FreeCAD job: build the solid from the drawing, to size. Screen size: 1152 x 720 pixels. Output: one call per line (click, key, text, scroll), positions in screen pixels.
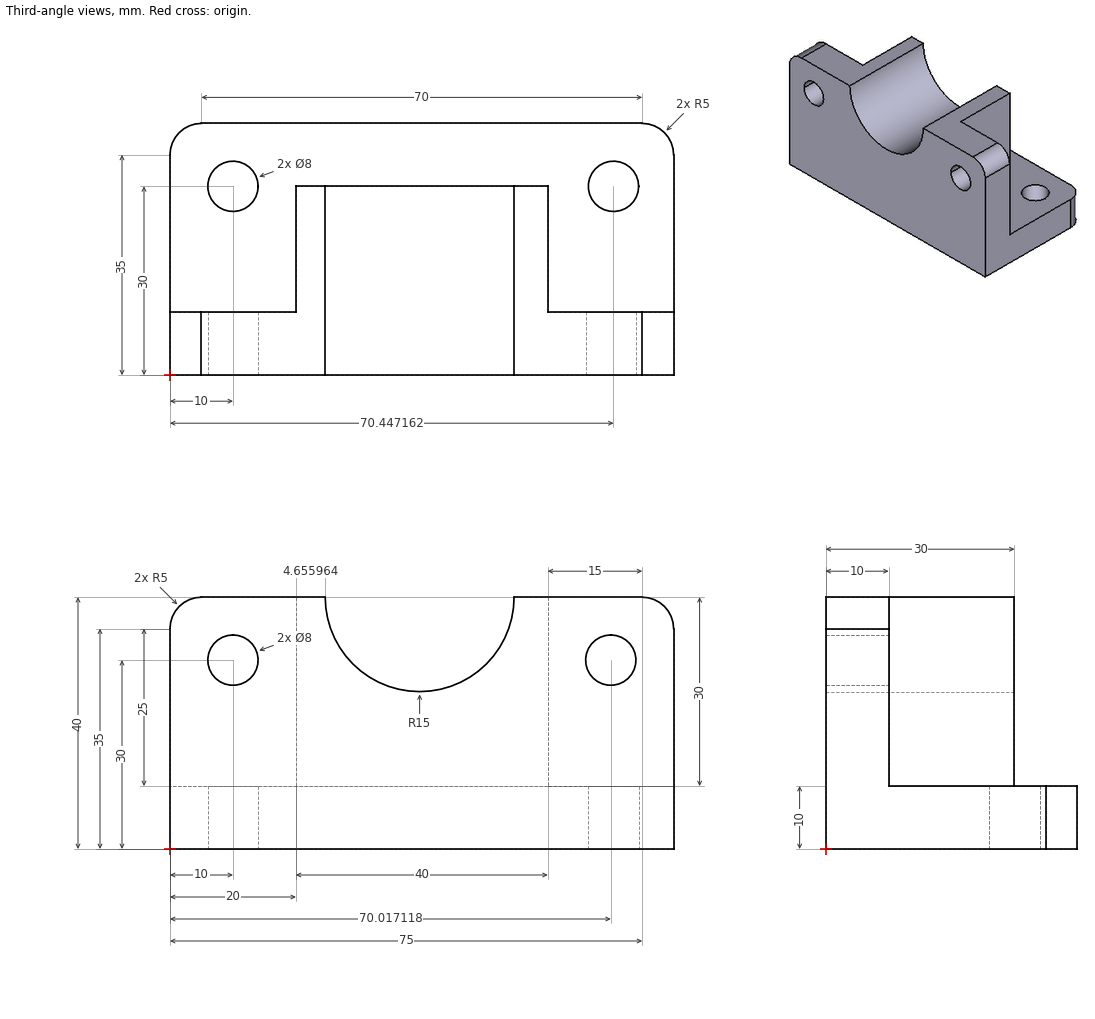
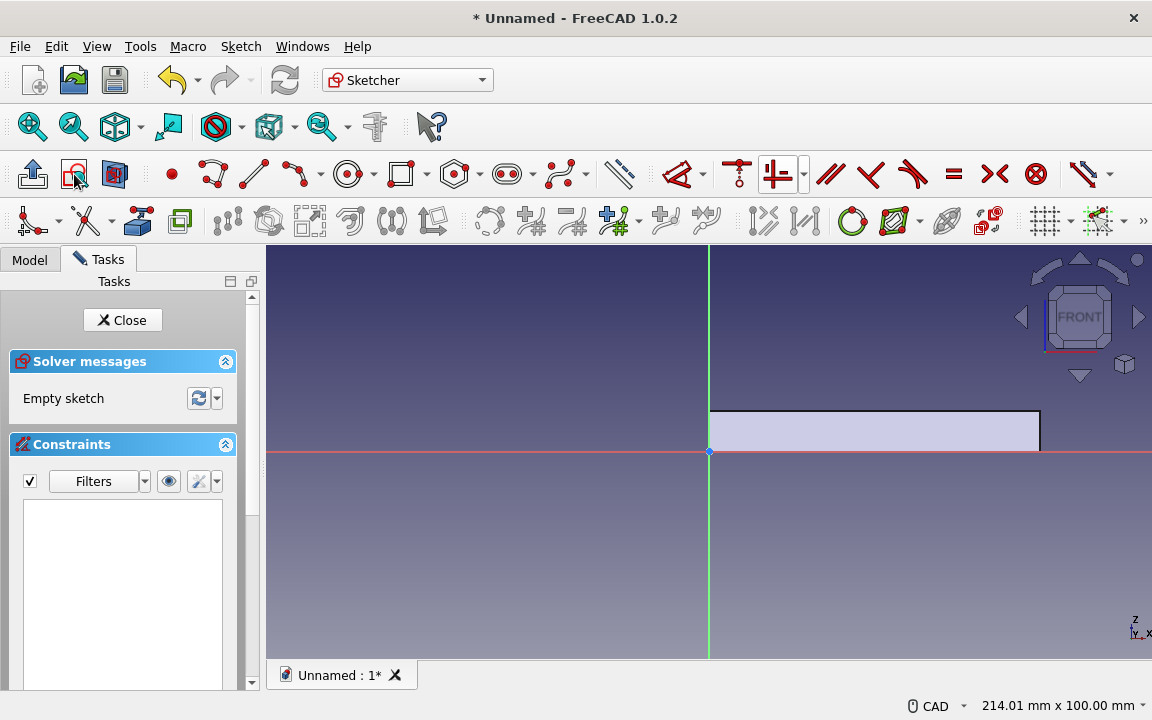
scroll(294, 631, down, 1)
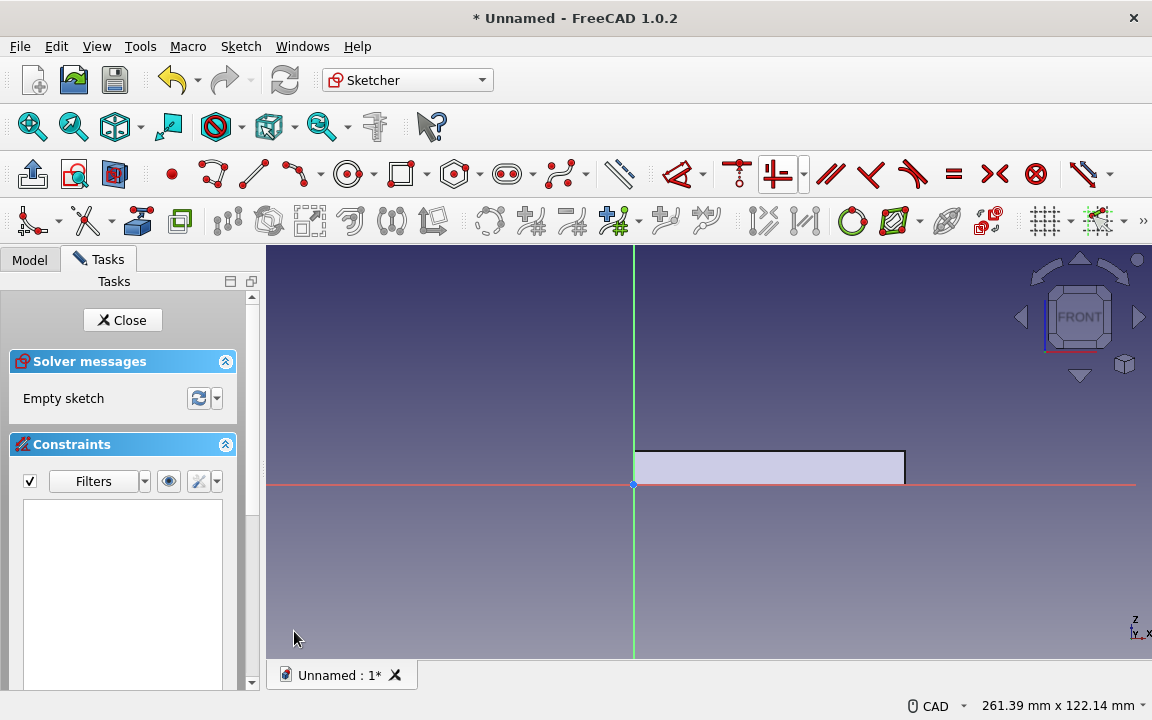
scroll(926, 374, up, 3)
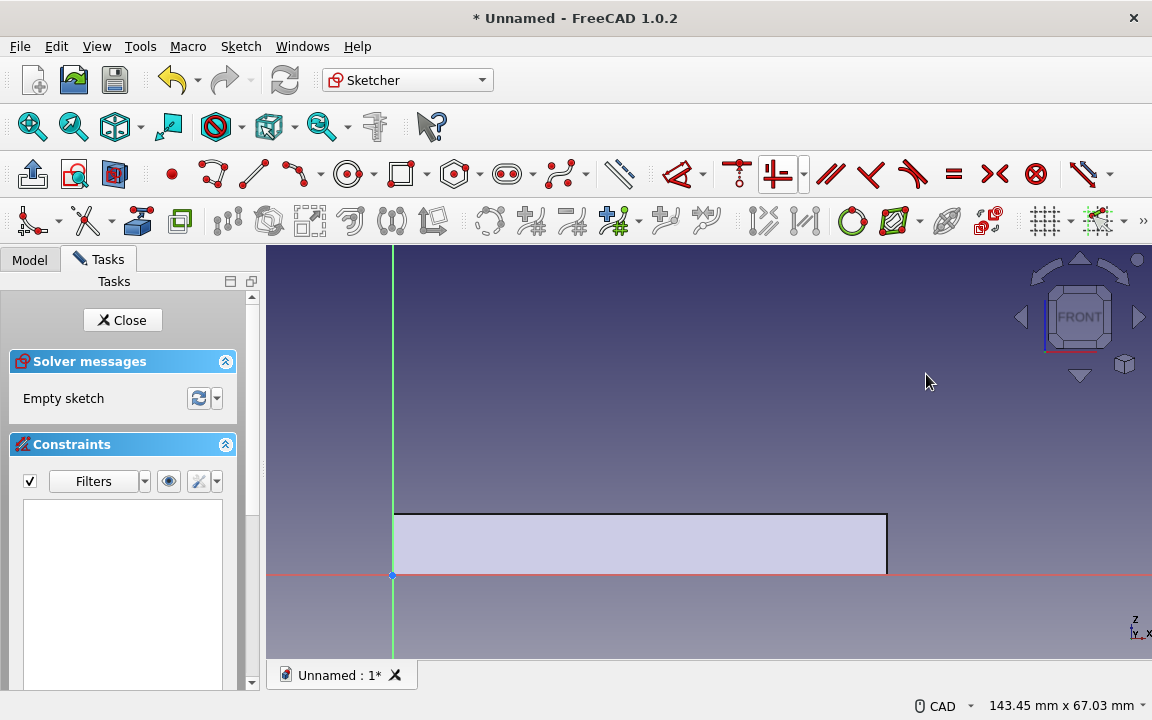
click(213, 174)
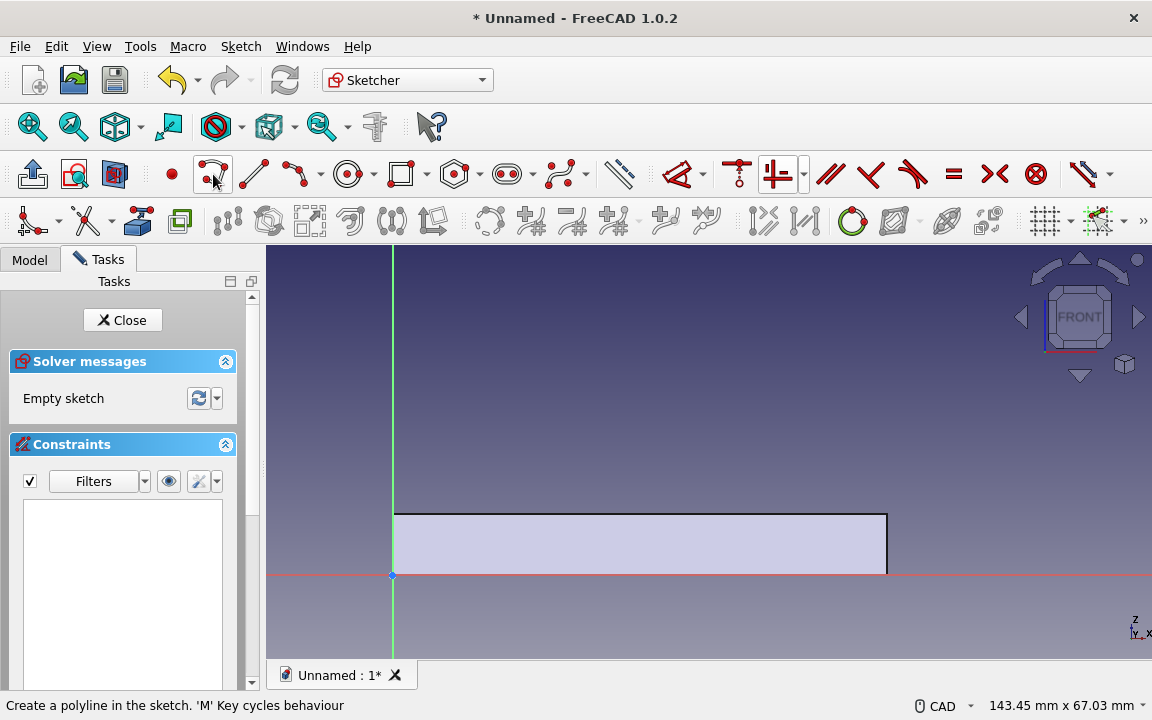
click(393, 359)
click(402, 514)
click(516, 514)
click(516, 328)
click(424, 328)
right_click(424, 328)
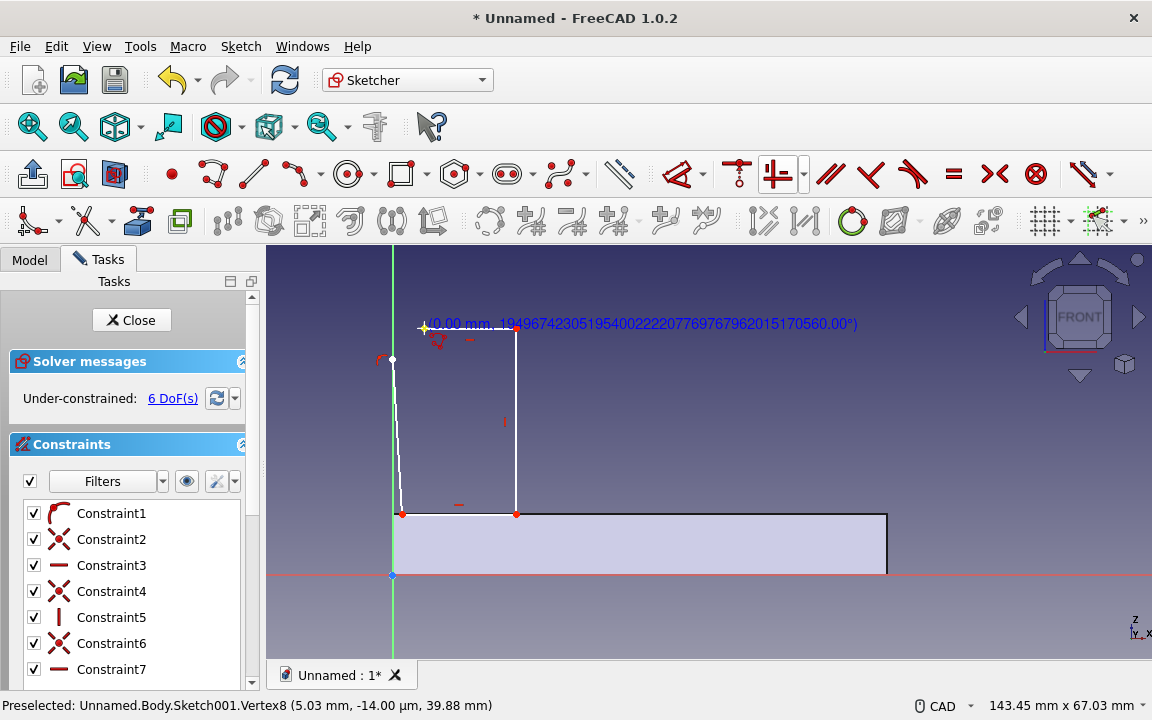
click(294, 174)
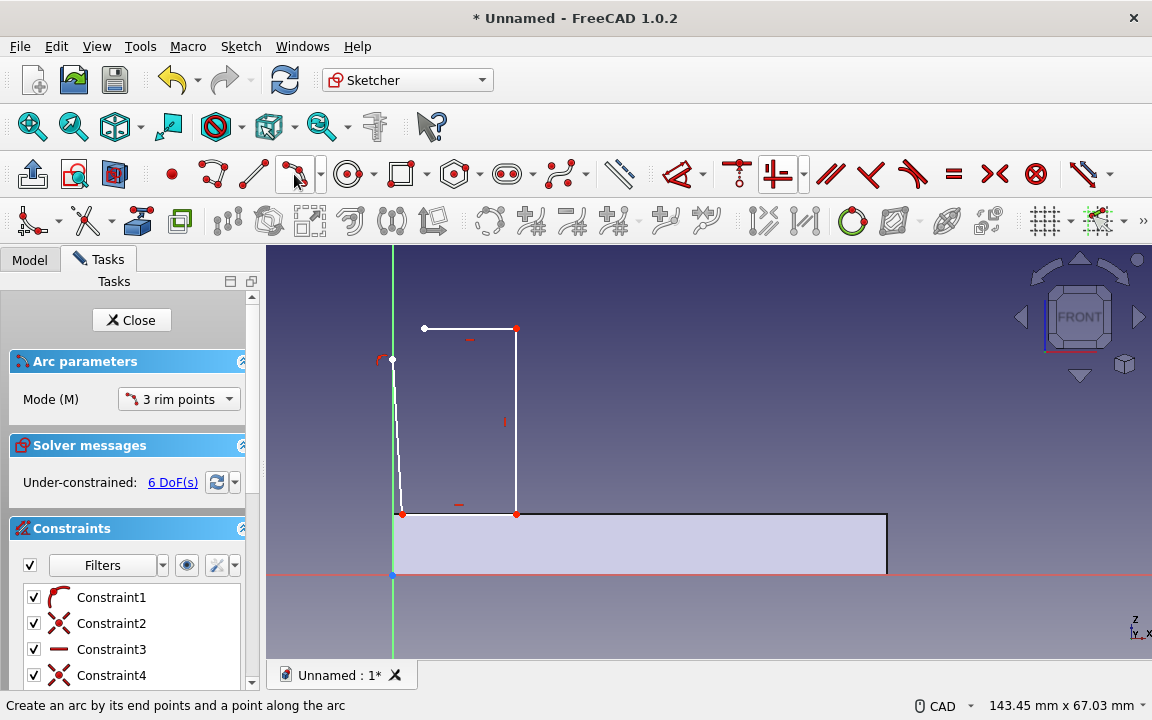
click(424, 329)
click(393, 360)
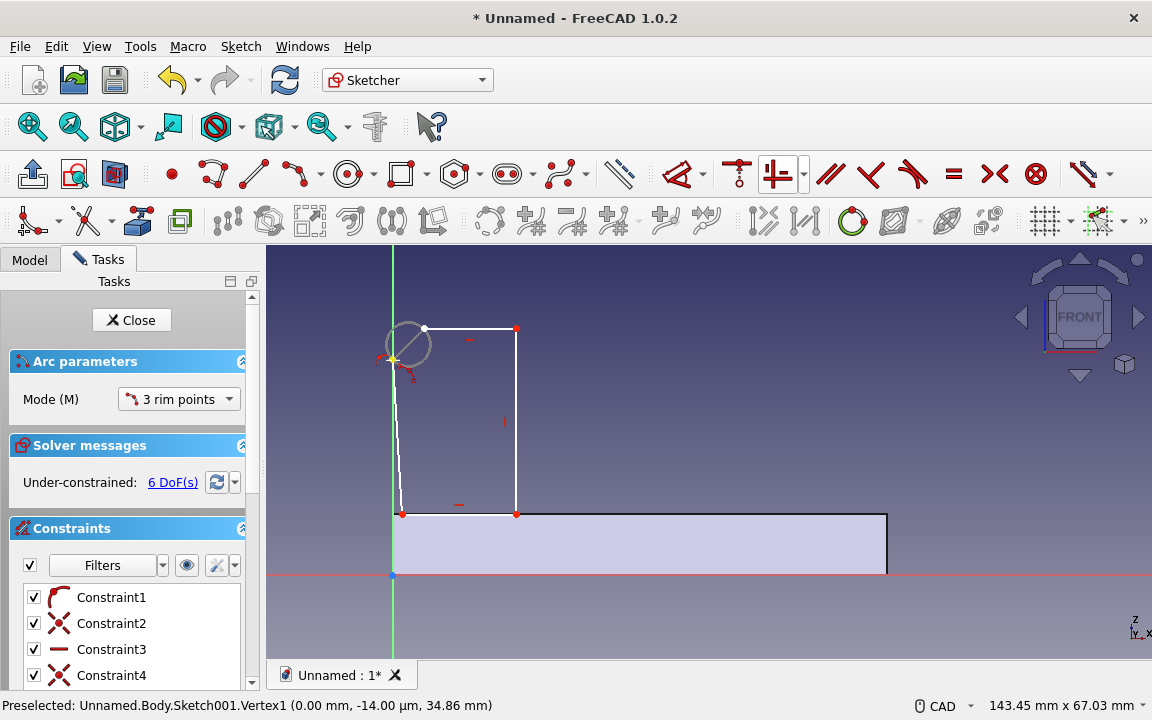
scroll(402, 337, up, 3)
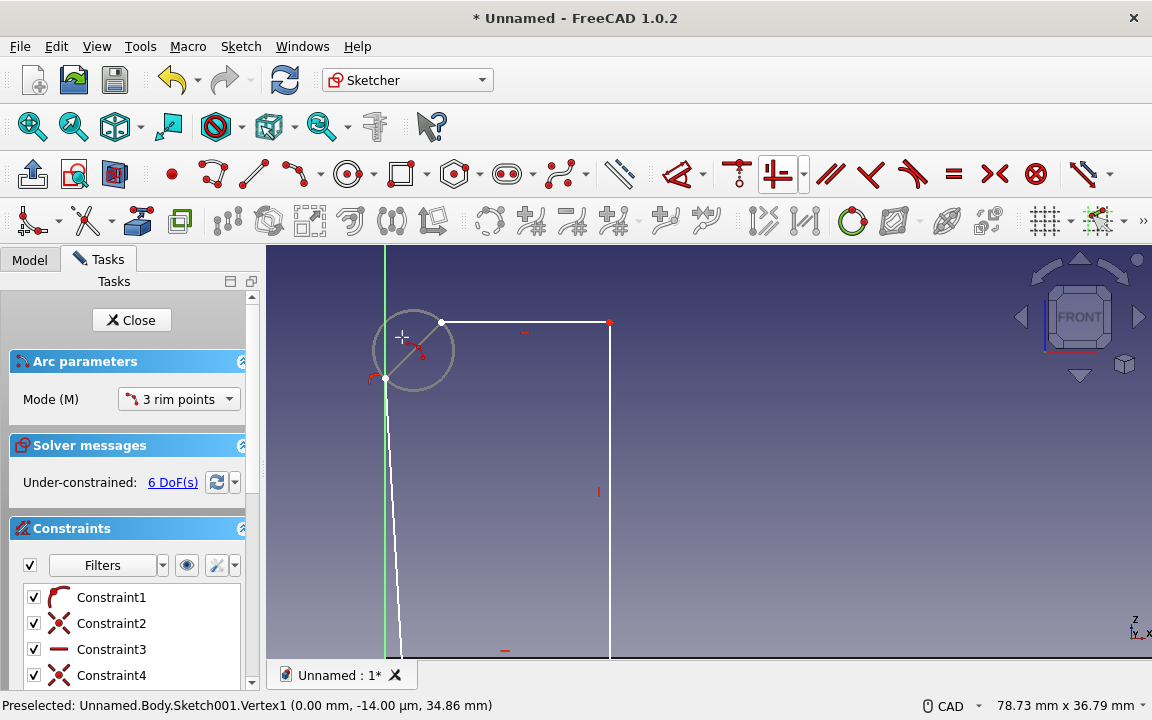
click(402, 337)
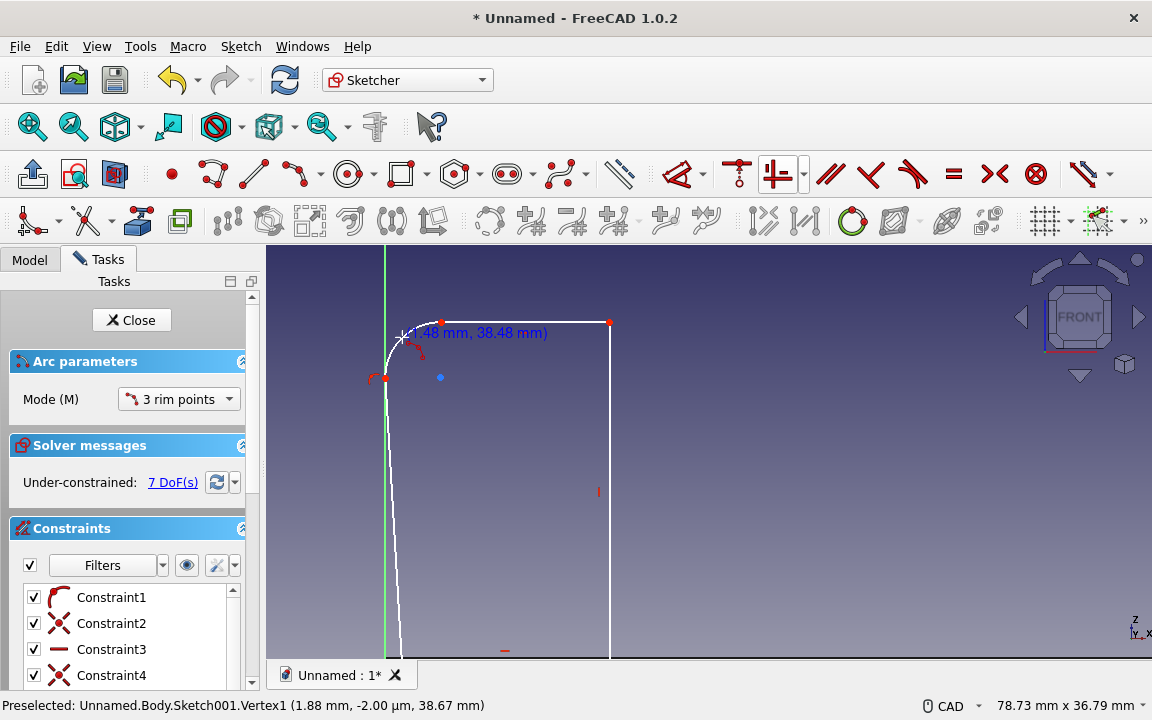
click(213, 174)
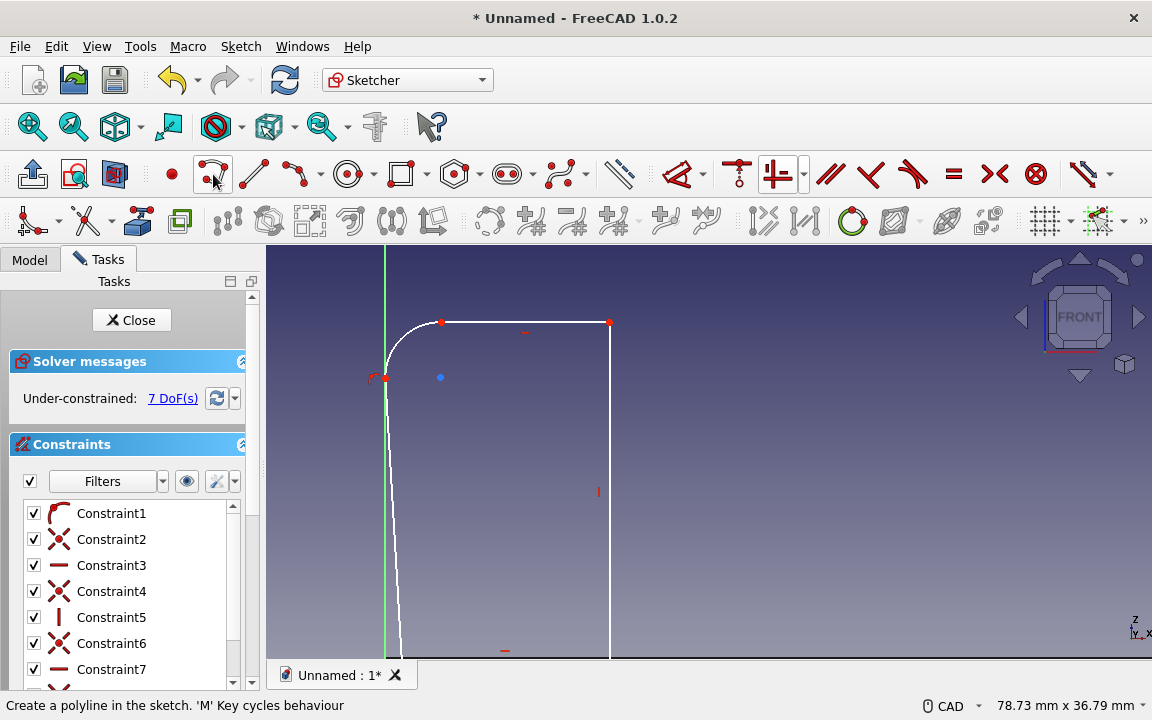
scroll(403, 338, down, 3)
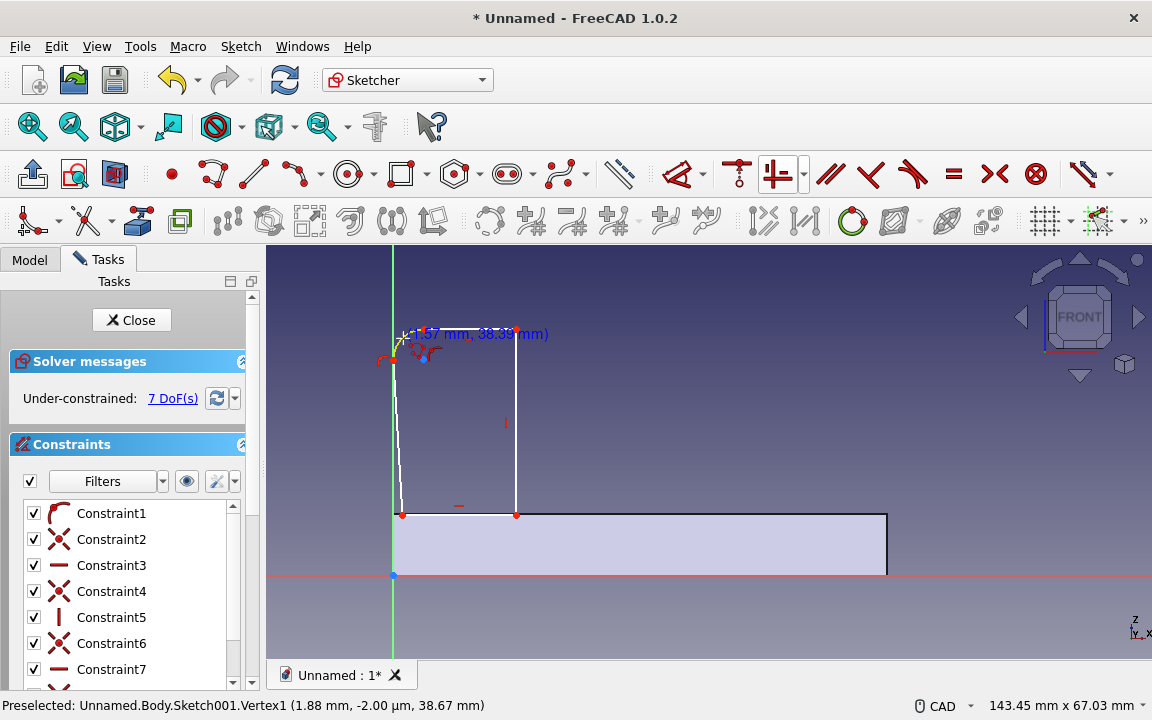
click(857, 329)
click(764, 329)
click(764, 514)
click(887, 514)
click(887, 360)
right_click(887, 360)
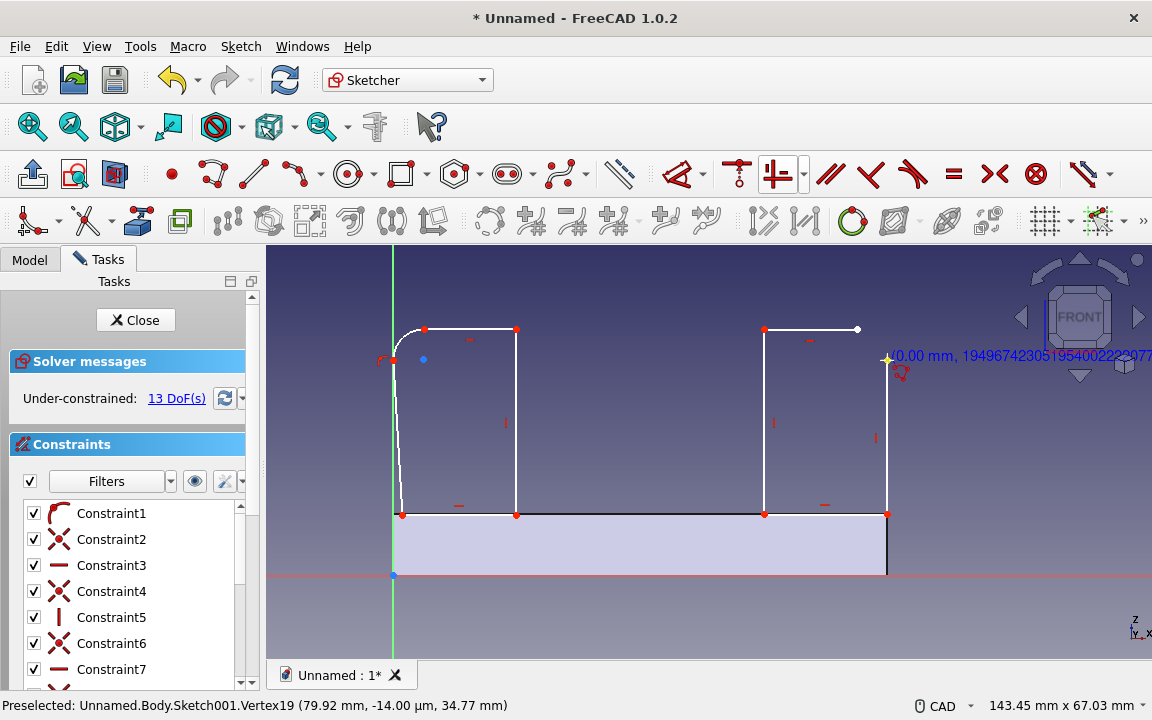
click(294, 174)